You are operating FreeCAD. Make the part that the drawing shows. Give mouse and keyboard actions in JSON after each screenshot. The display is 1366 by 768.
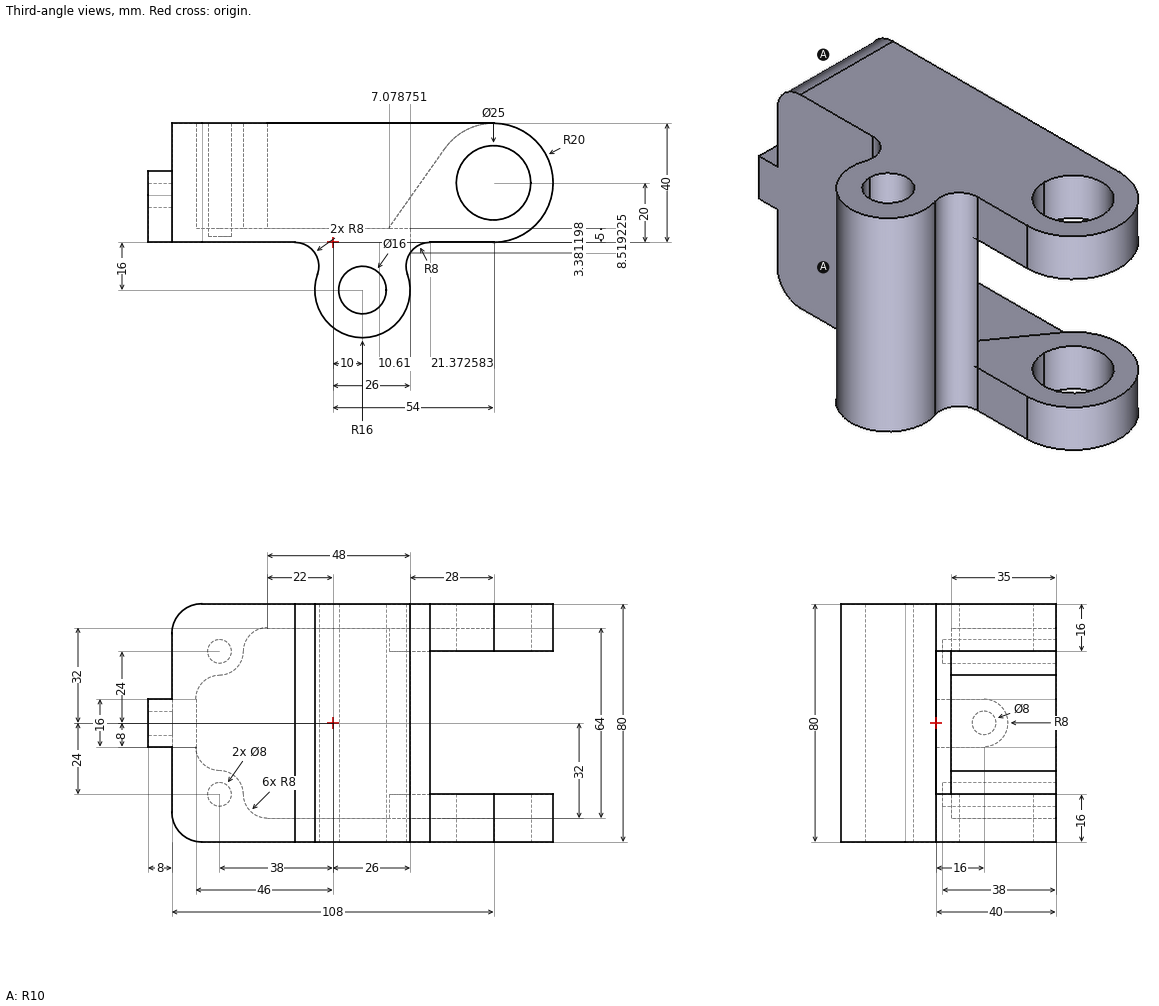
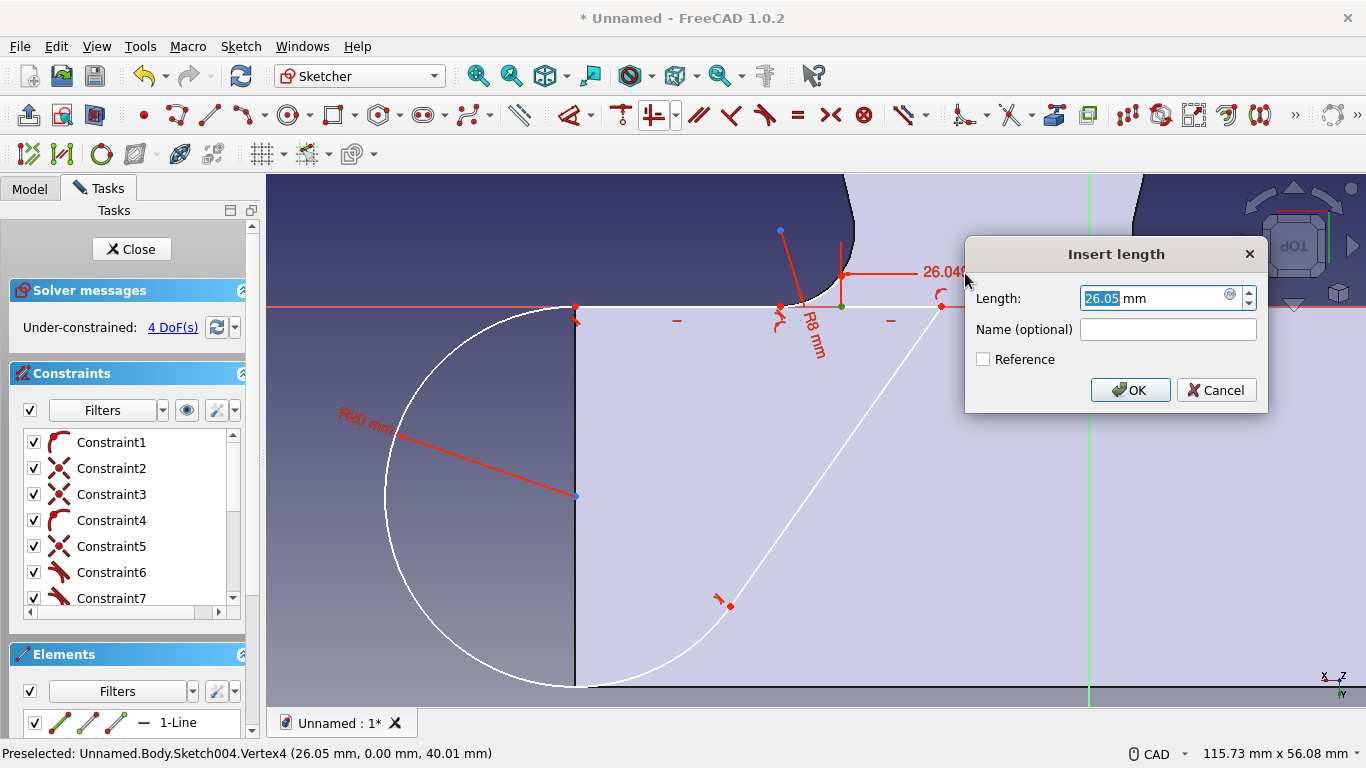
{"action": "type", "text": "26"}
{"action": "key", "text": "Return"}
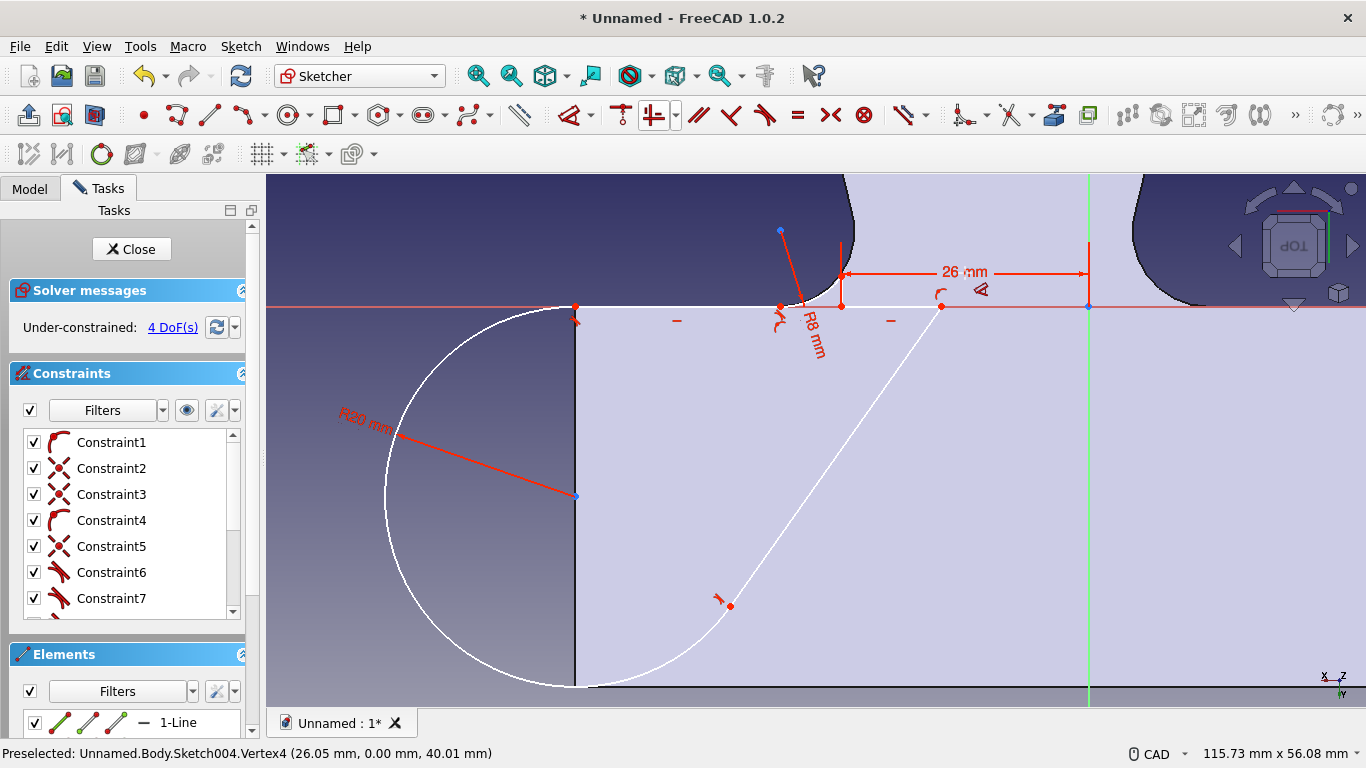
{"action": "left_click", "coordinate": [575, 307]}
{"action": "left_click", "coordinate": [714, 273]}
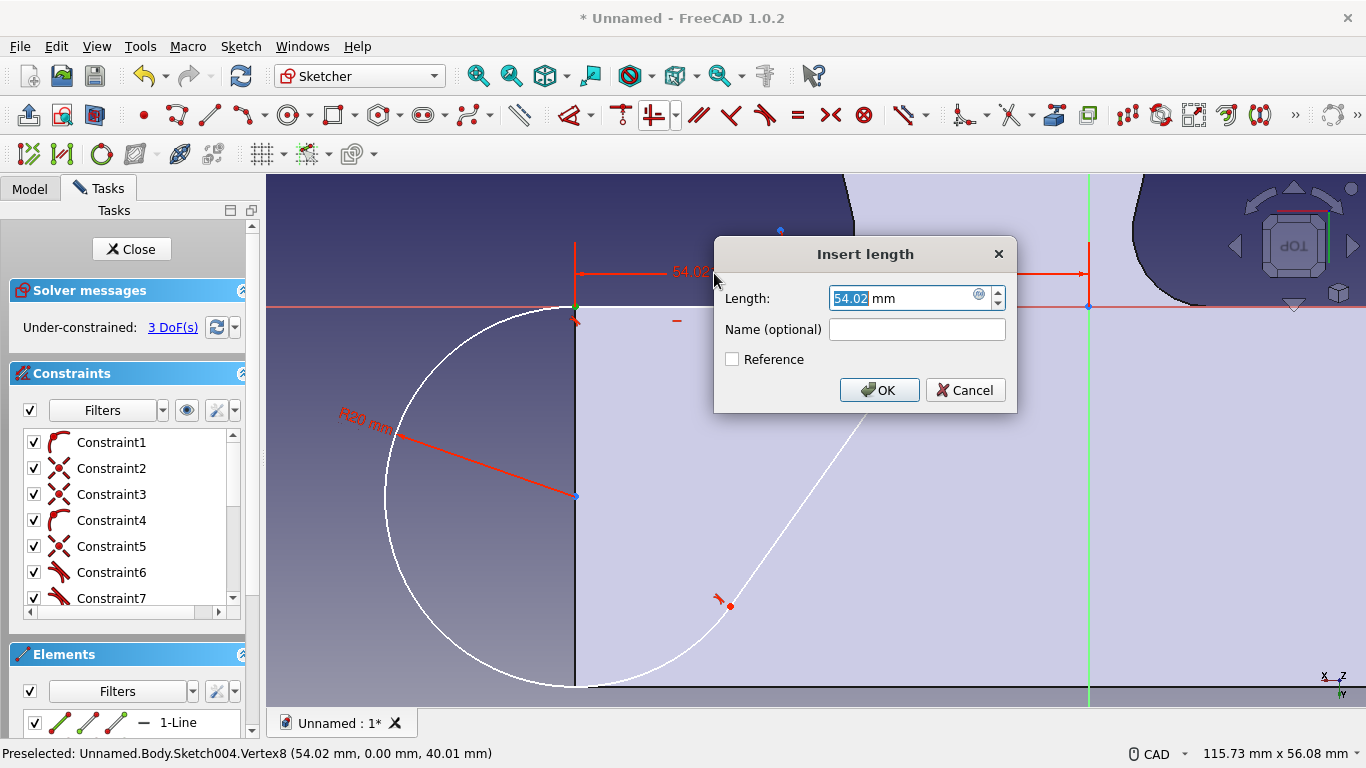
{"action": "type", "text": "54"}
{"action": "key", "text": "Return"}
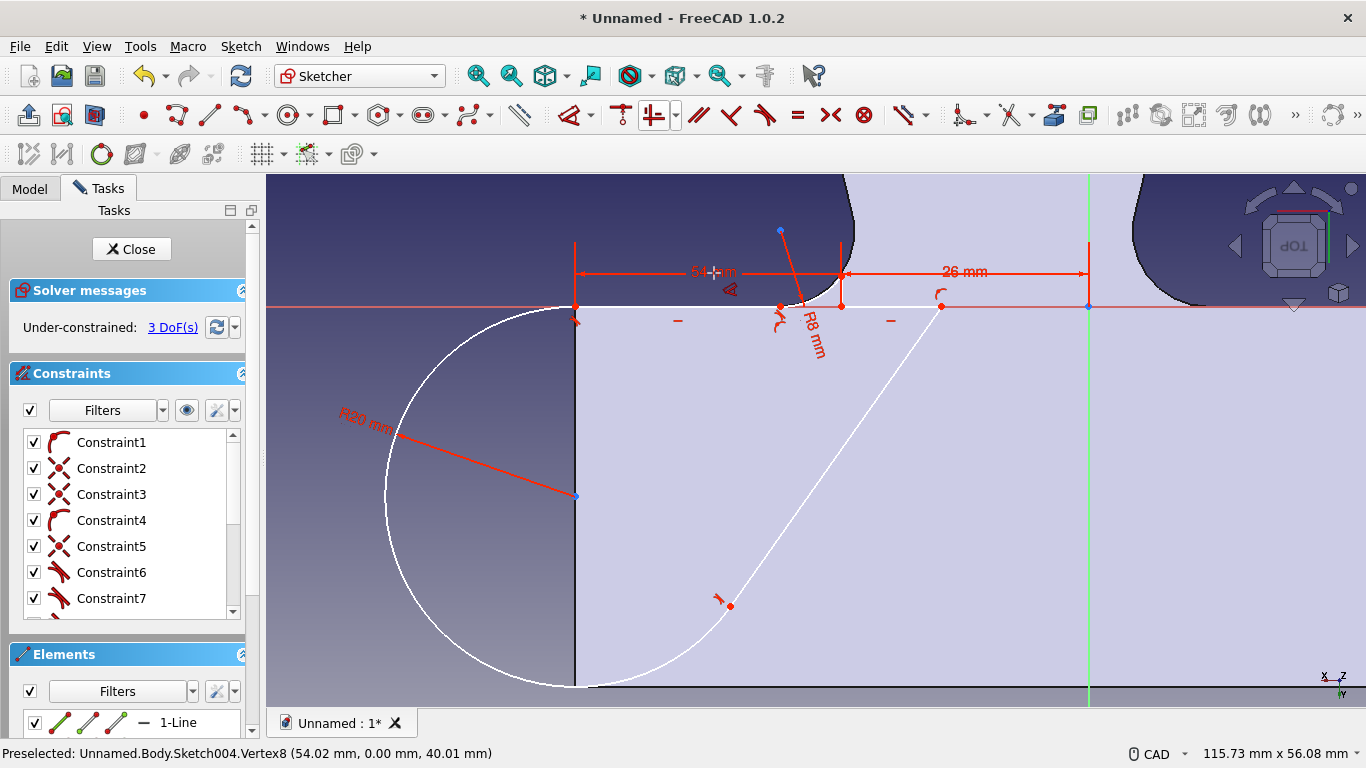
{"action": "left_click", "coordinate": [912, 307]}
{"action": "left_click", "coordinate": [892, 273]}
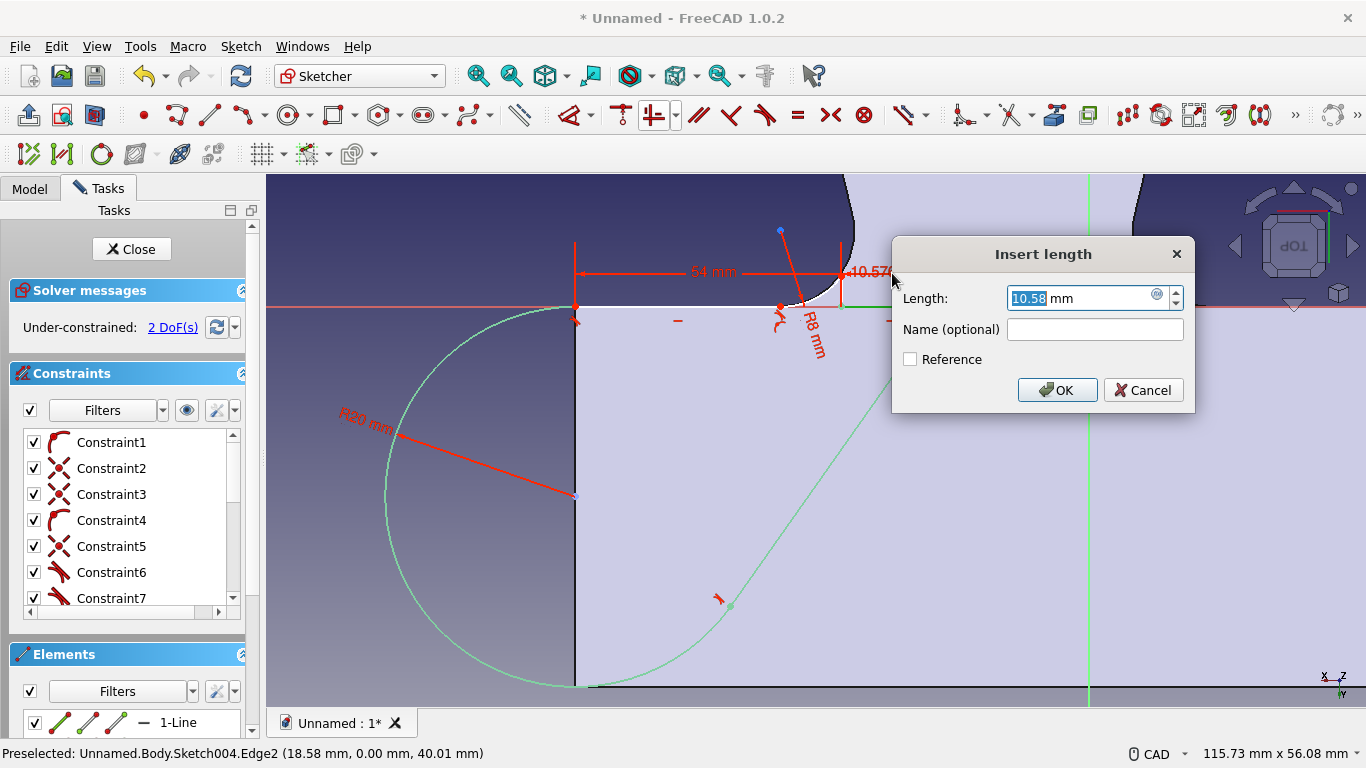
{"action": "type", "text": "10.61"}
{"action": "key", "text": "Return"}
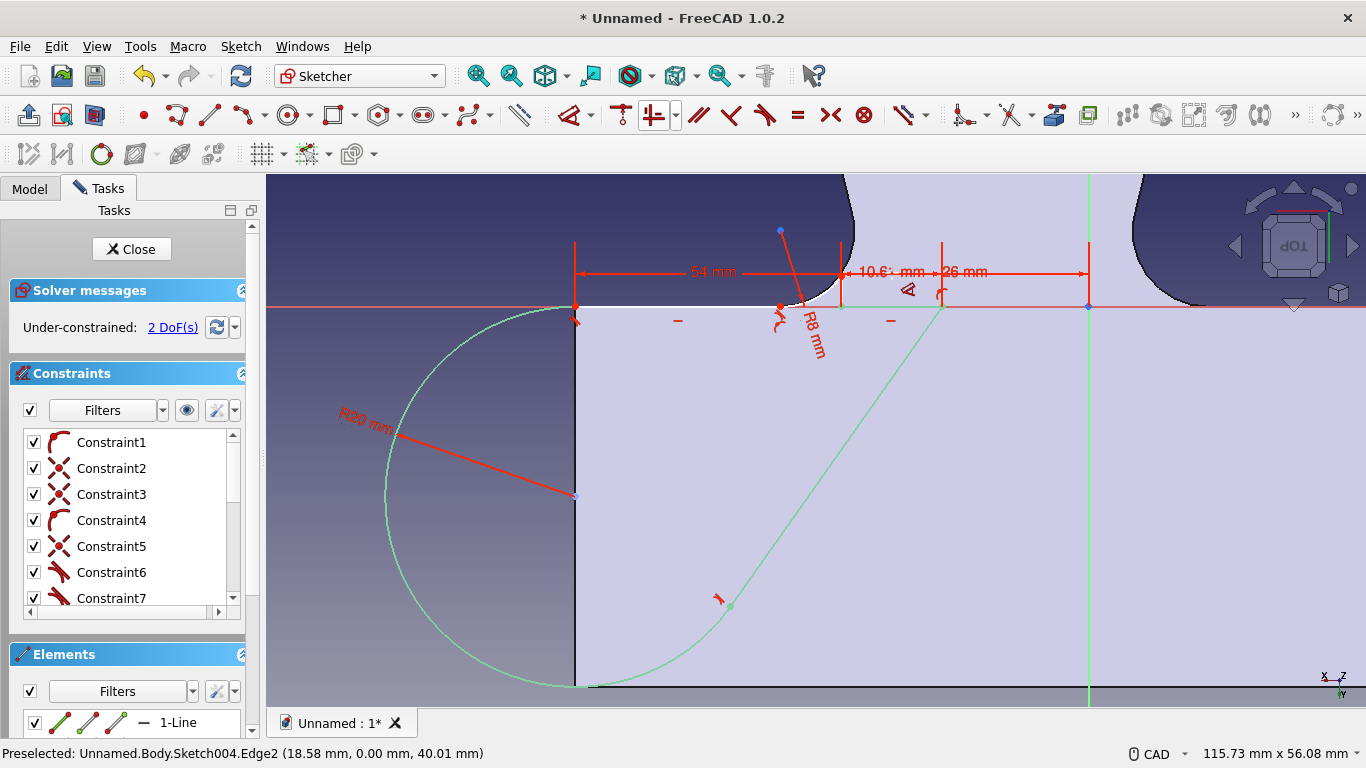
{"action": "left_click", "coordinate": [719, 307]}
{"action": "left_click", "coordinate": [631, 273]}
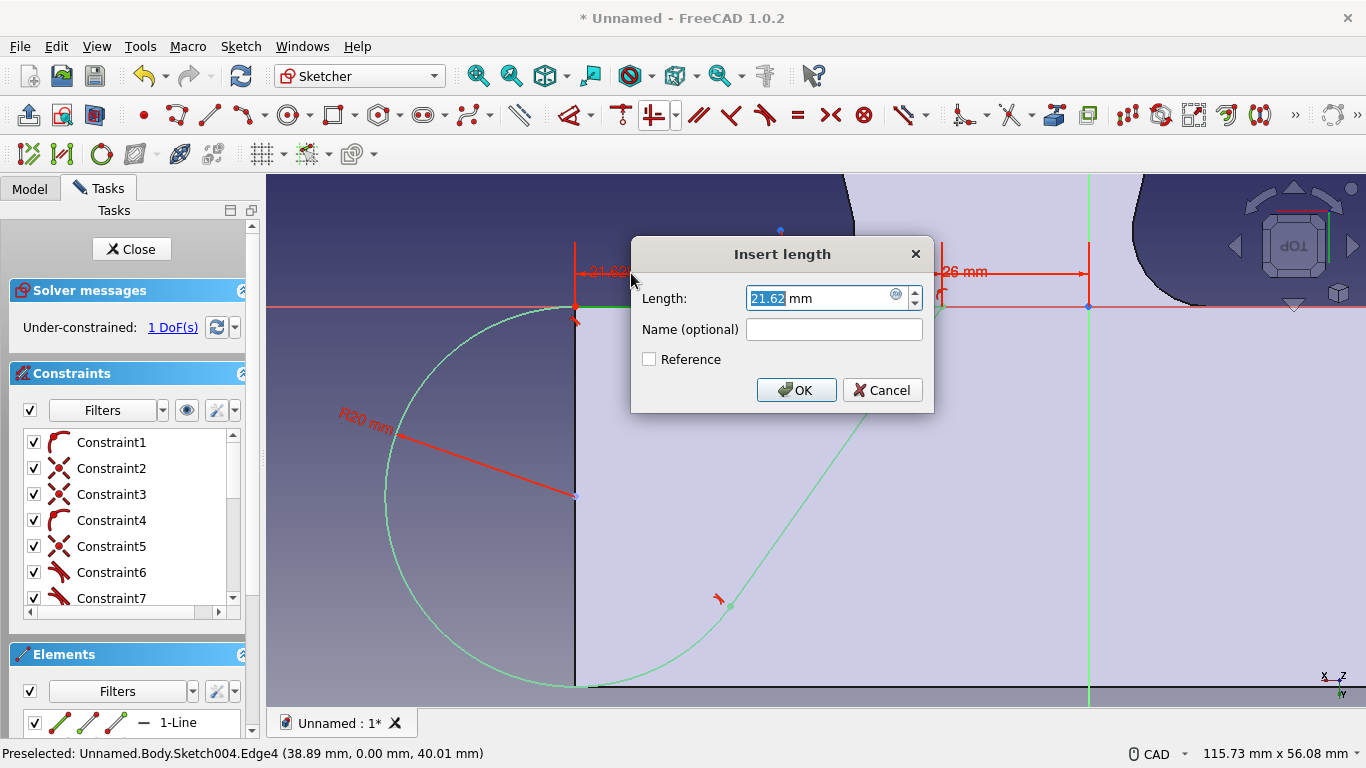
{"action": "type", "text": "21.372583"}
{"action": "key", "text": "Return"}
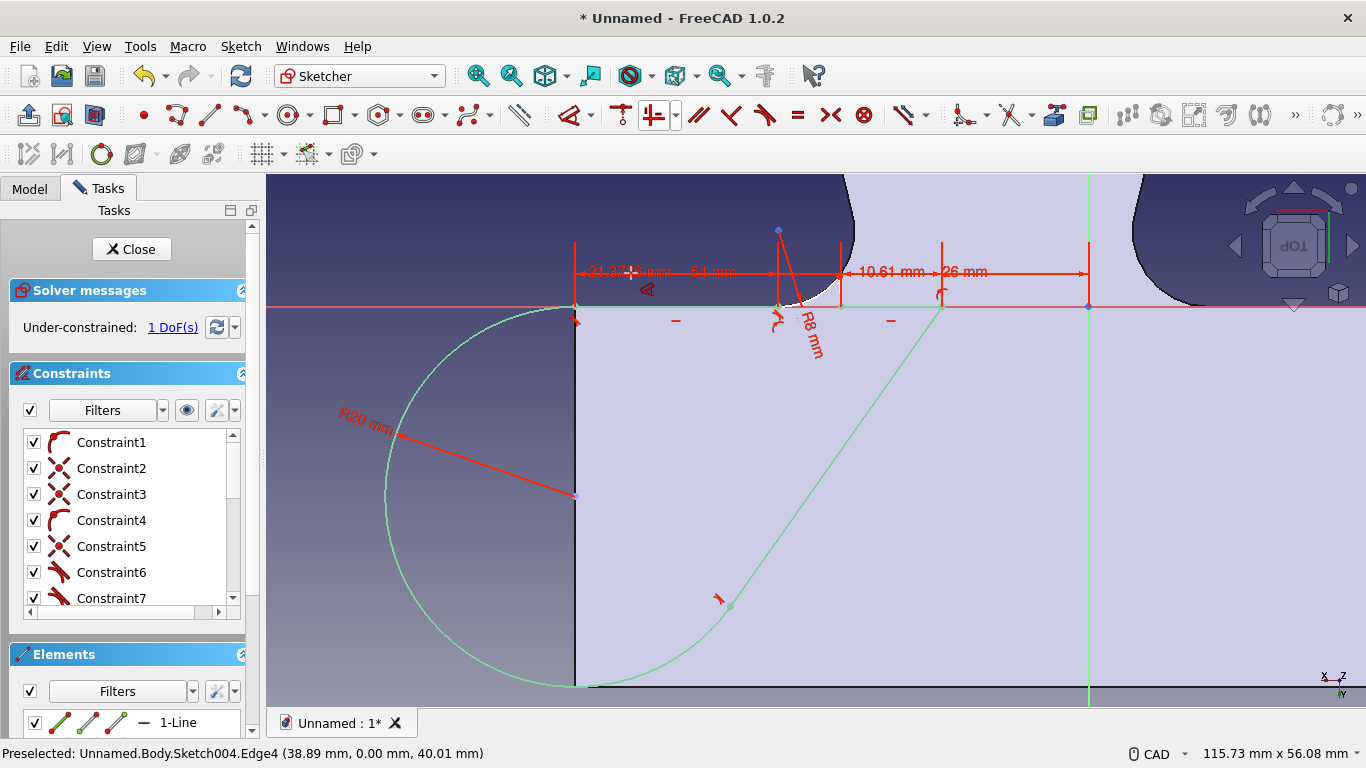
{"action": "scroll", "coordinate": [839, 276], "scroll_direction": "up", "scroll_amount": 2}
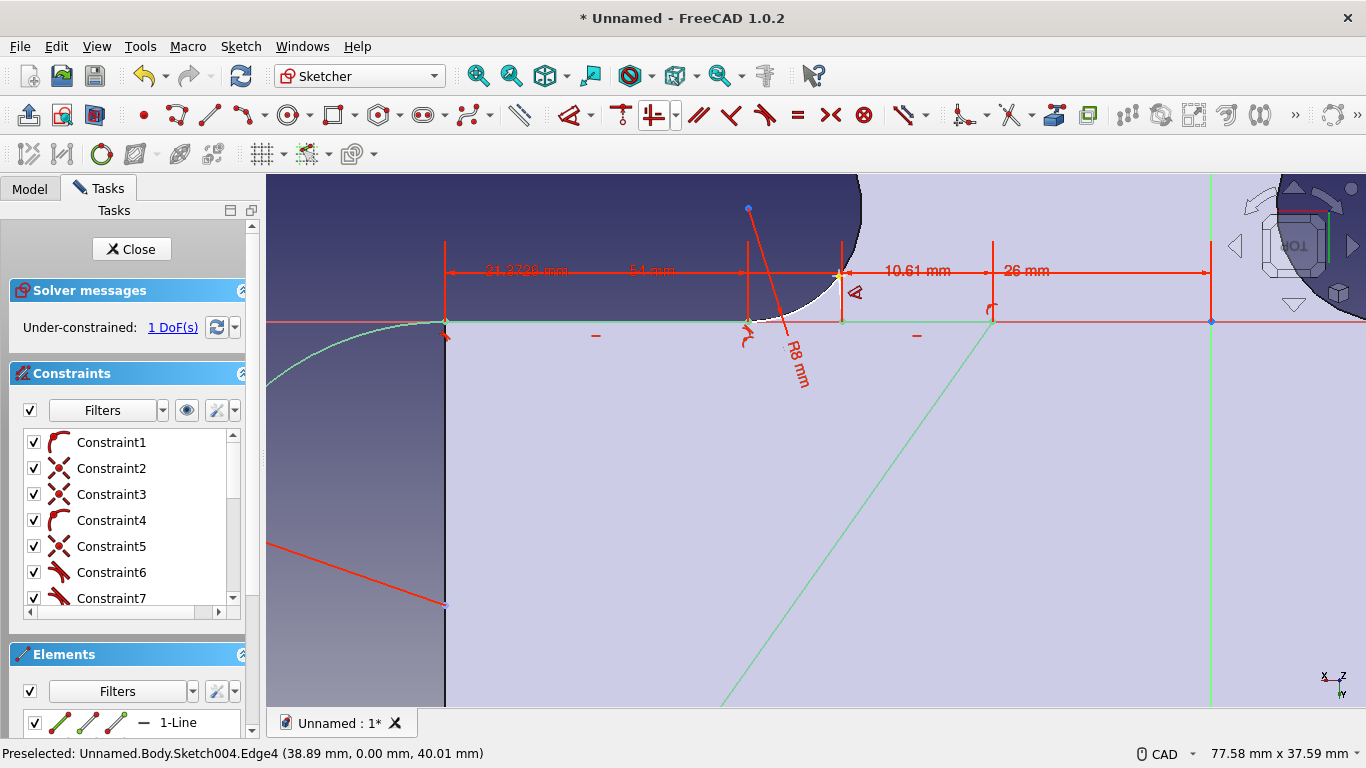
{"action": "left_click", "coordinate": [839, 277]}
{"action": "left_click", "coordinate": [805, 289]}